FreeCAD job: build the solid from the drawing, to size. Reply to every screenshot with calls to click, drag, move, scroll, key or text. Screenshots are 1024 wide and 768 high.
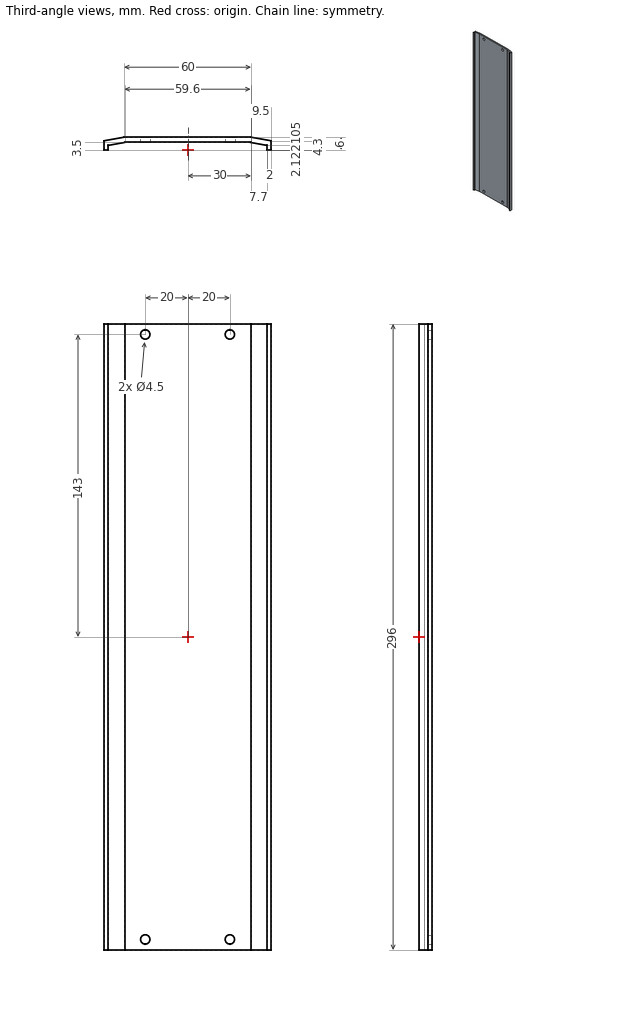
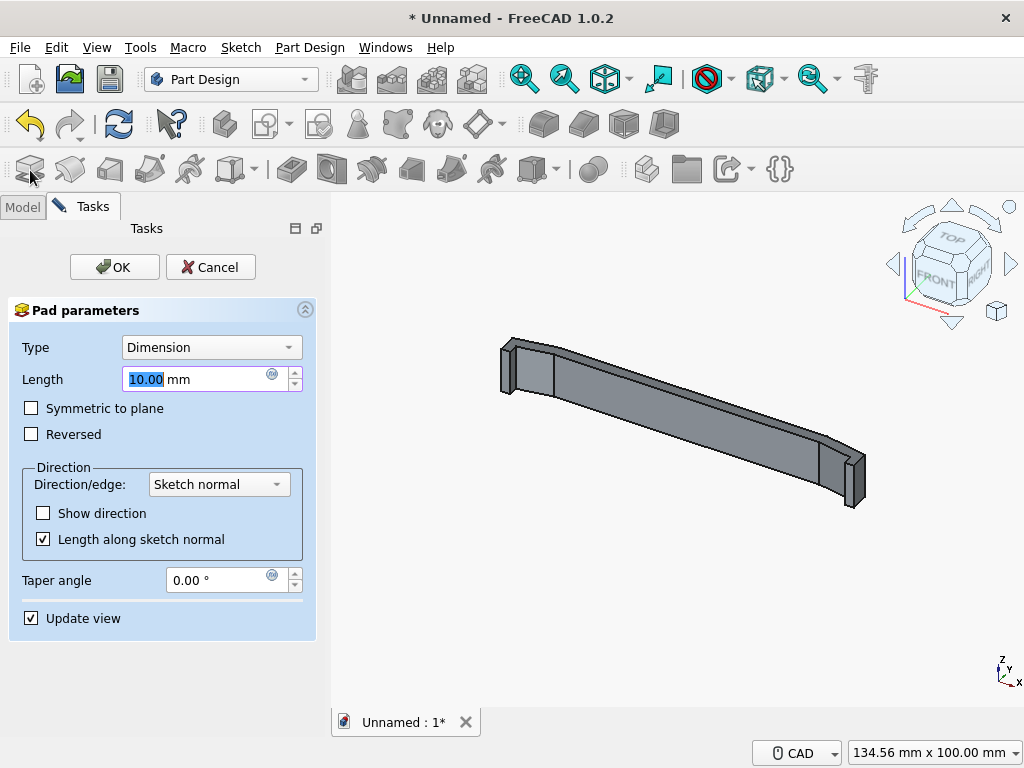
text(296)
key(Tab)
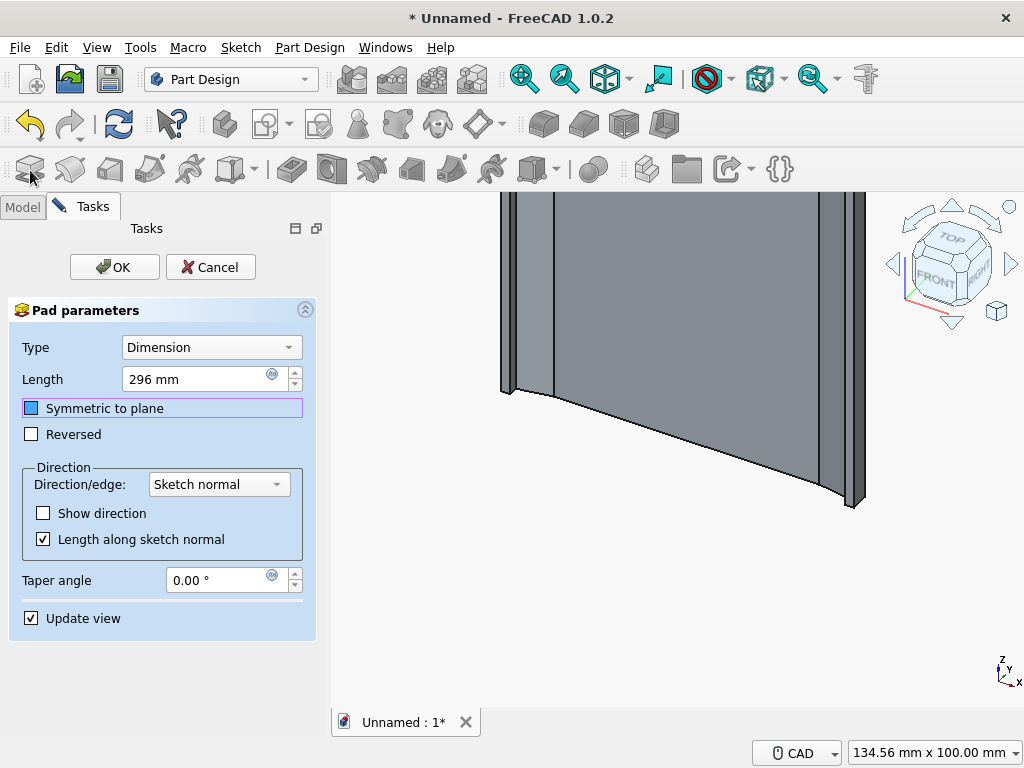
click(30, 408)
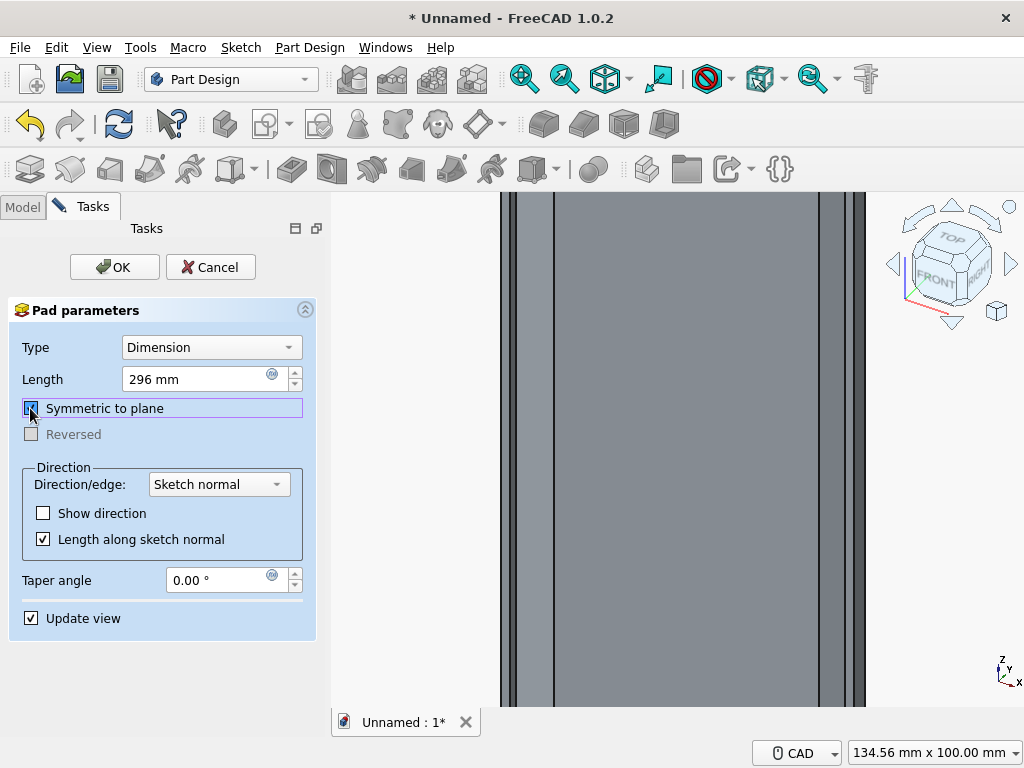
click(115, 267)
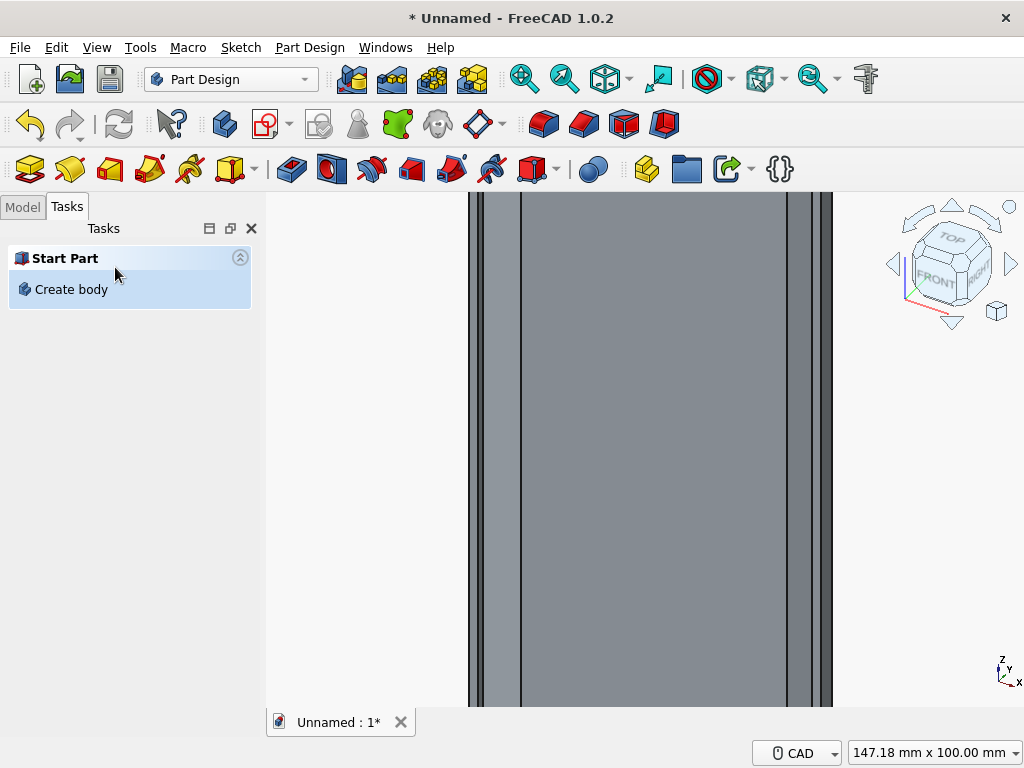
key(v)
key(f)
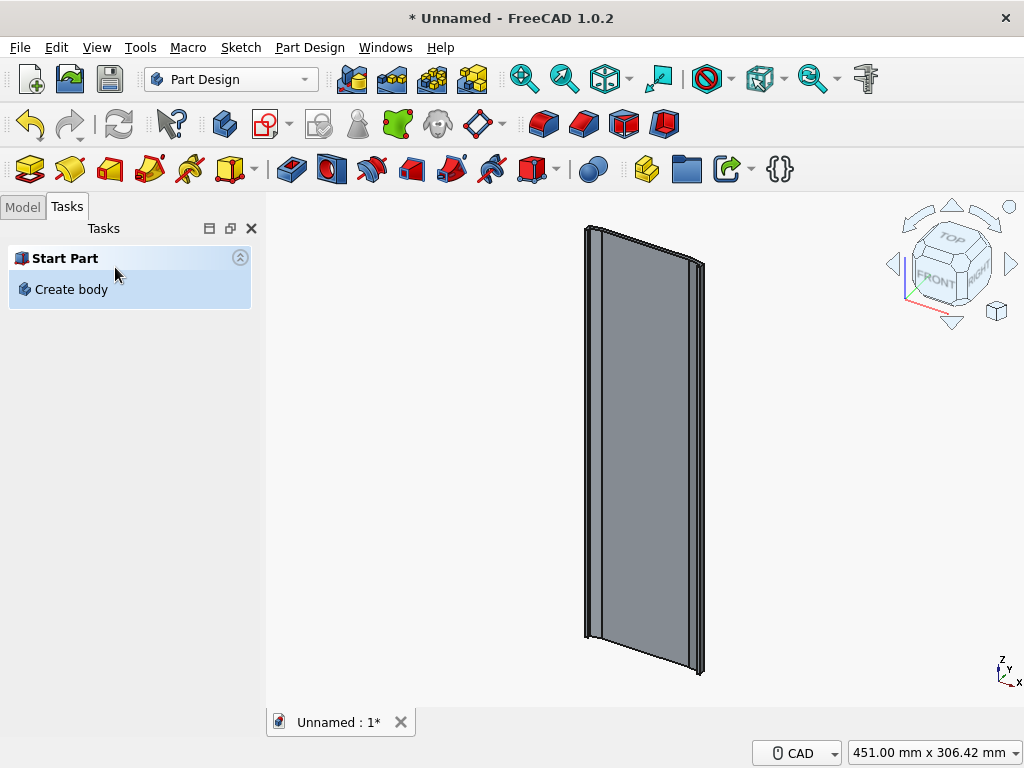
key(4)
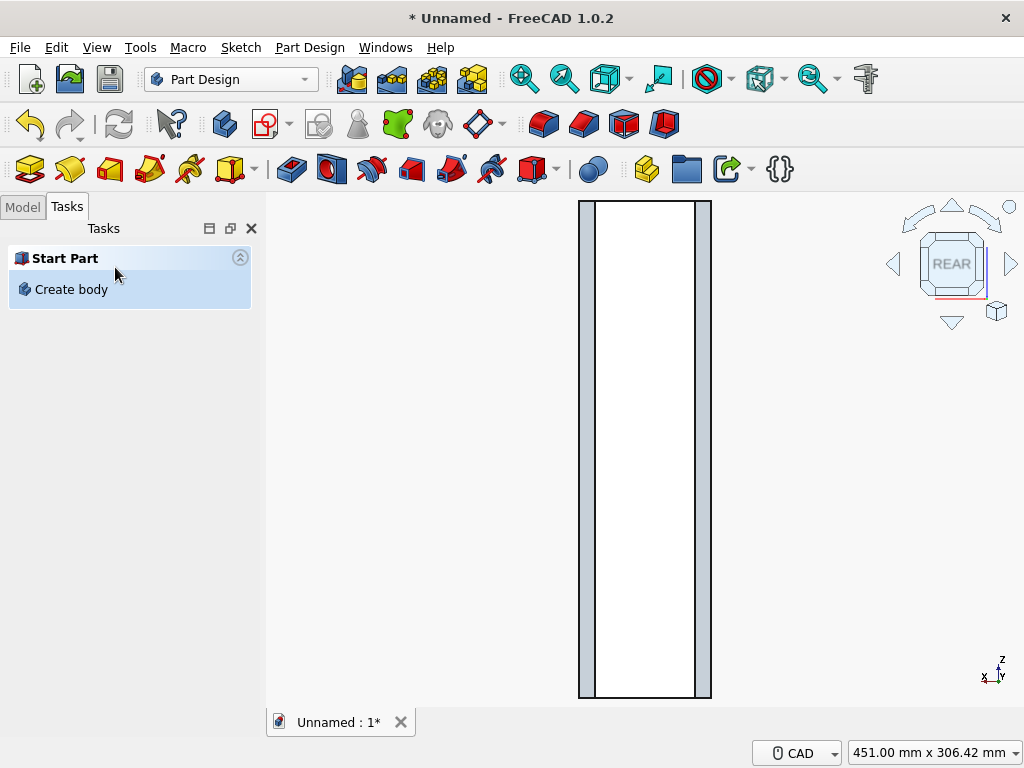
click(645, 306)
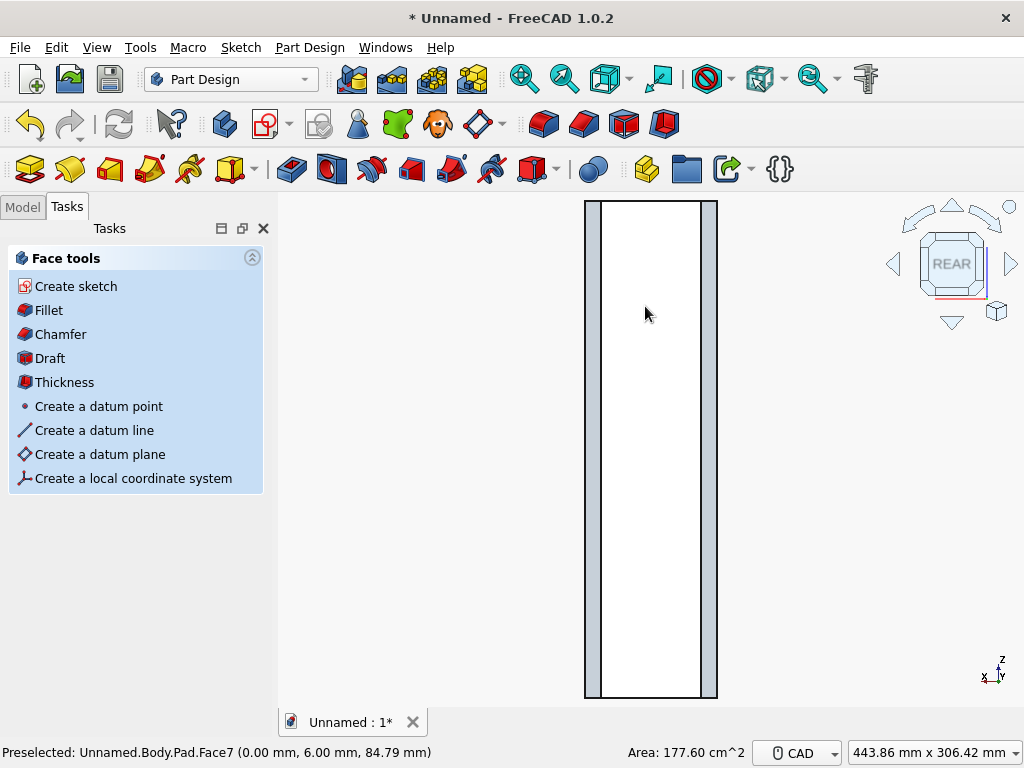
click(266, 124)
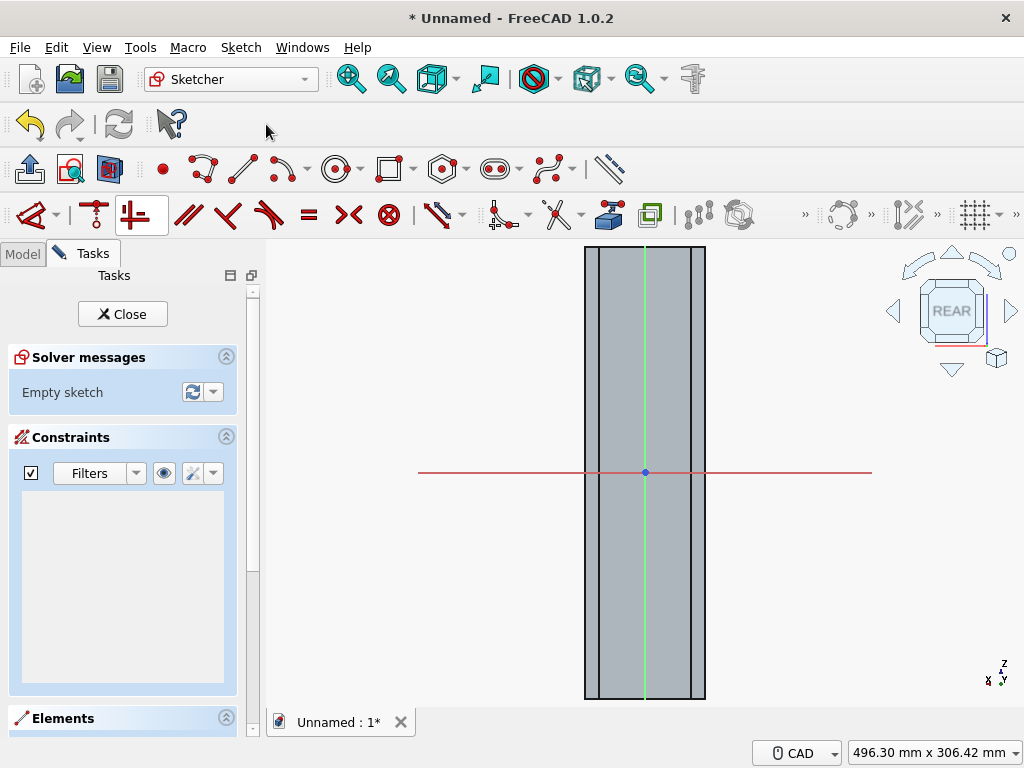
scroll(576, 473, down, 5)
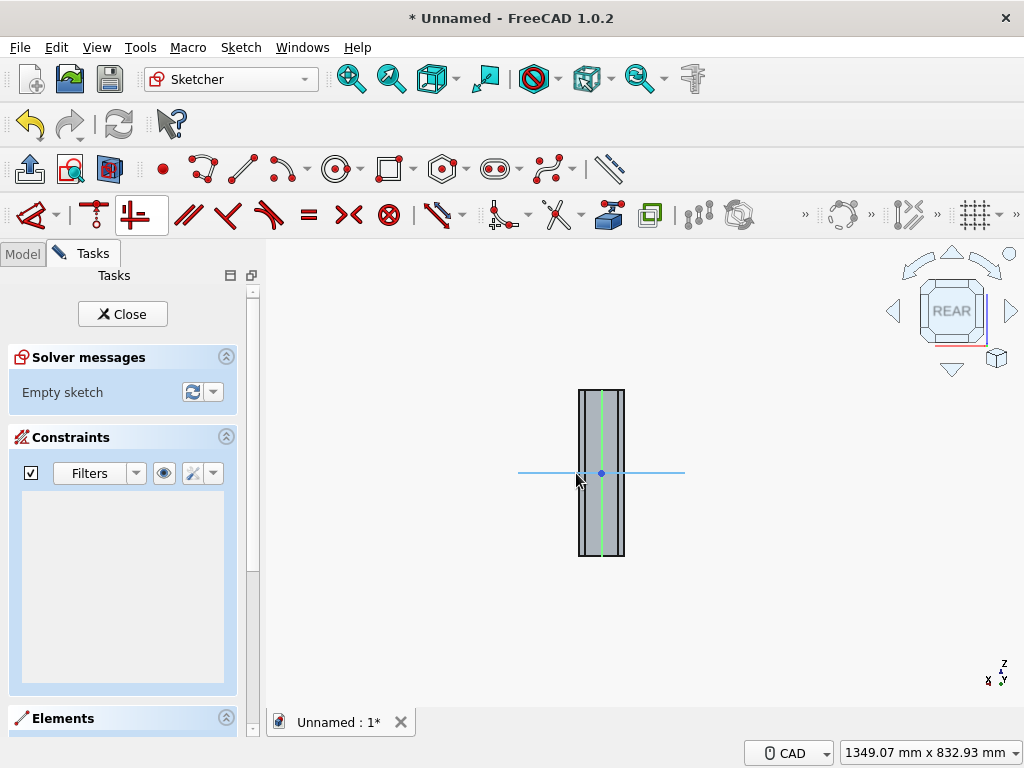
scroll(603, 388, up, 14)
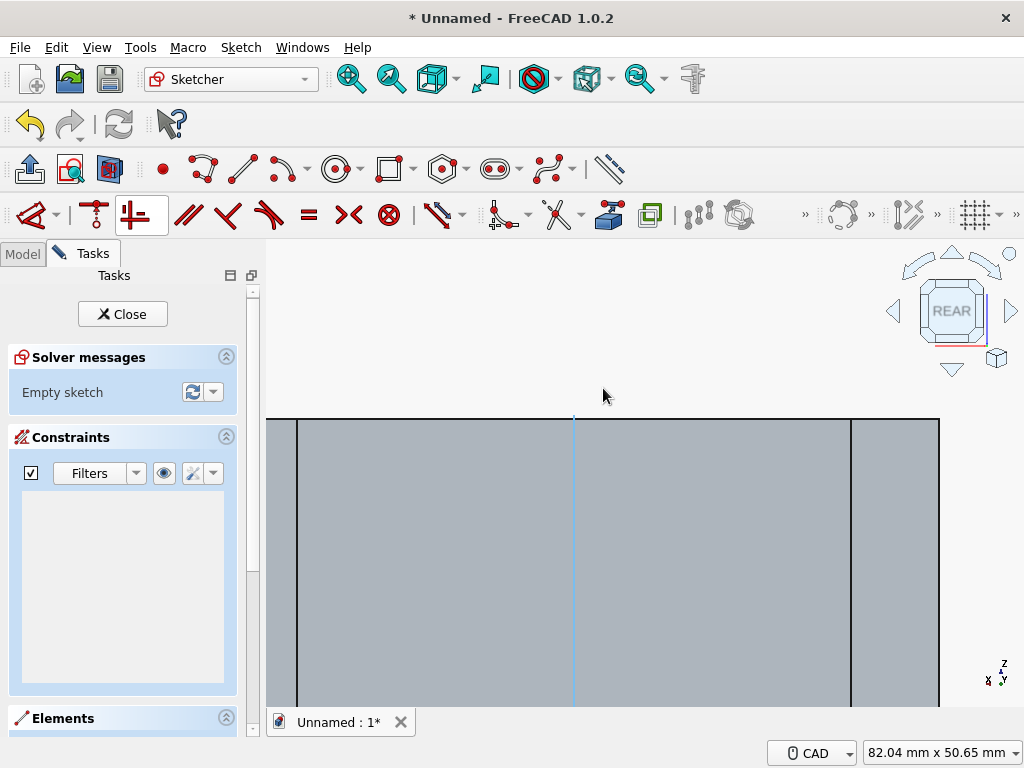
click(336, 170)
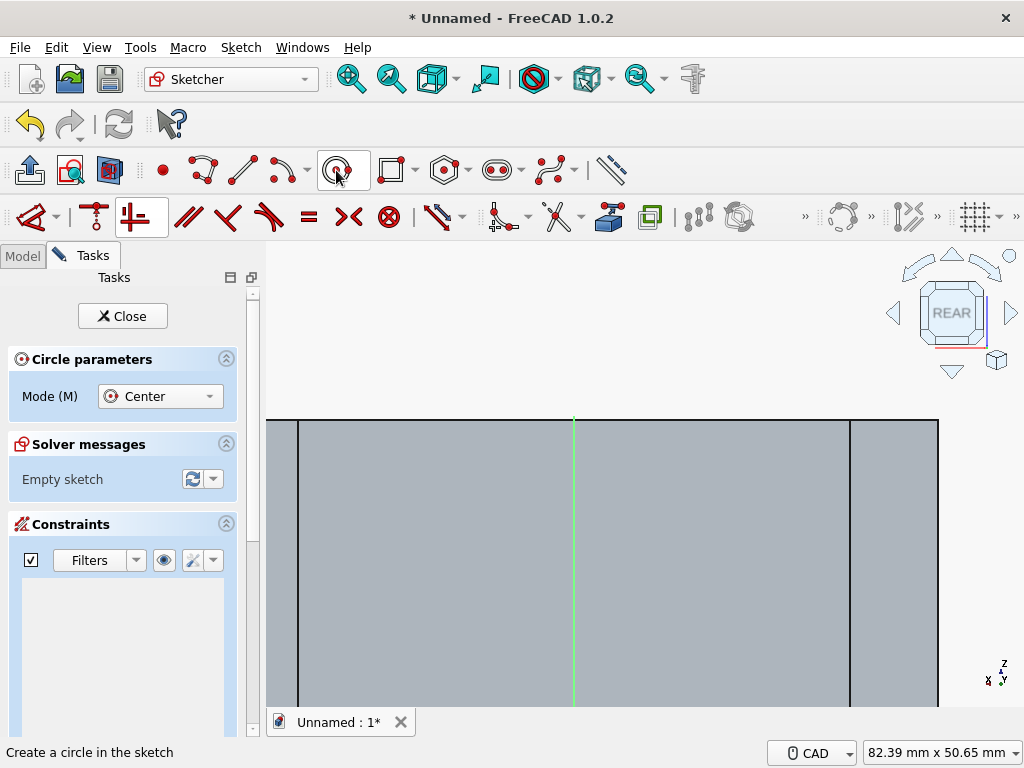
click(758, 466)
move(773, 451)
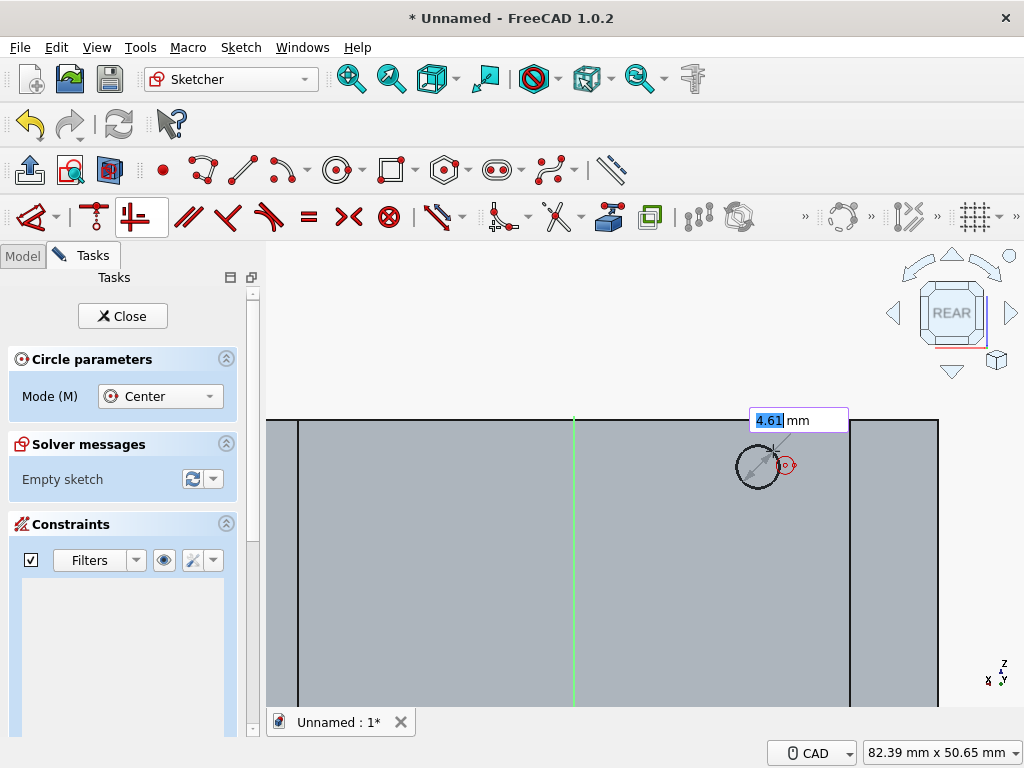
text(4.5)
key(Return)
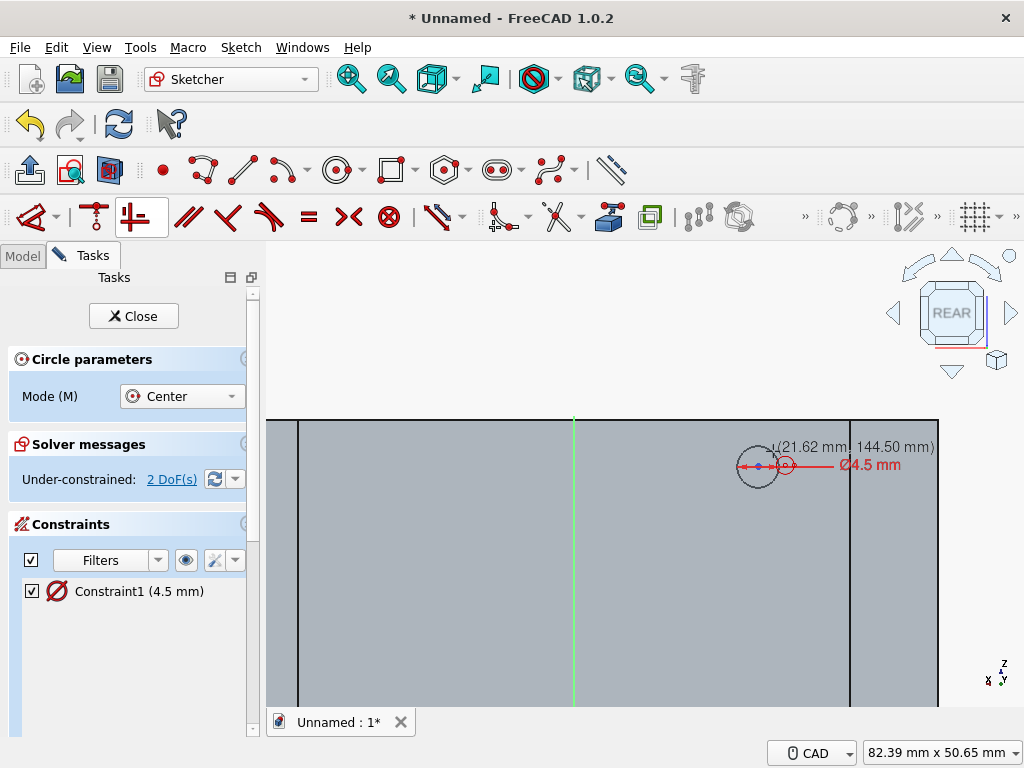
click(390, 466)
move(405, 451)